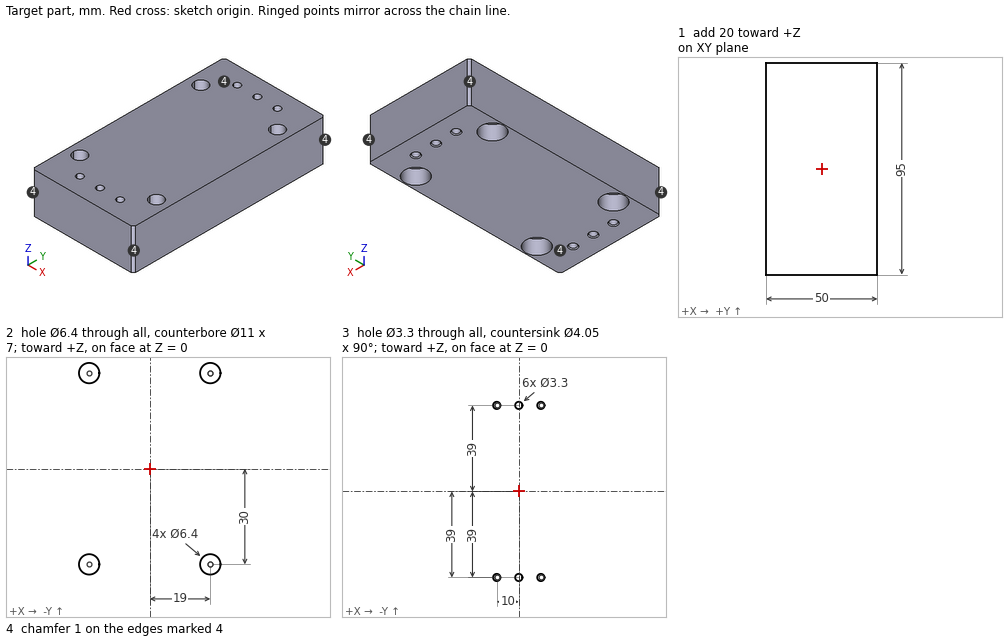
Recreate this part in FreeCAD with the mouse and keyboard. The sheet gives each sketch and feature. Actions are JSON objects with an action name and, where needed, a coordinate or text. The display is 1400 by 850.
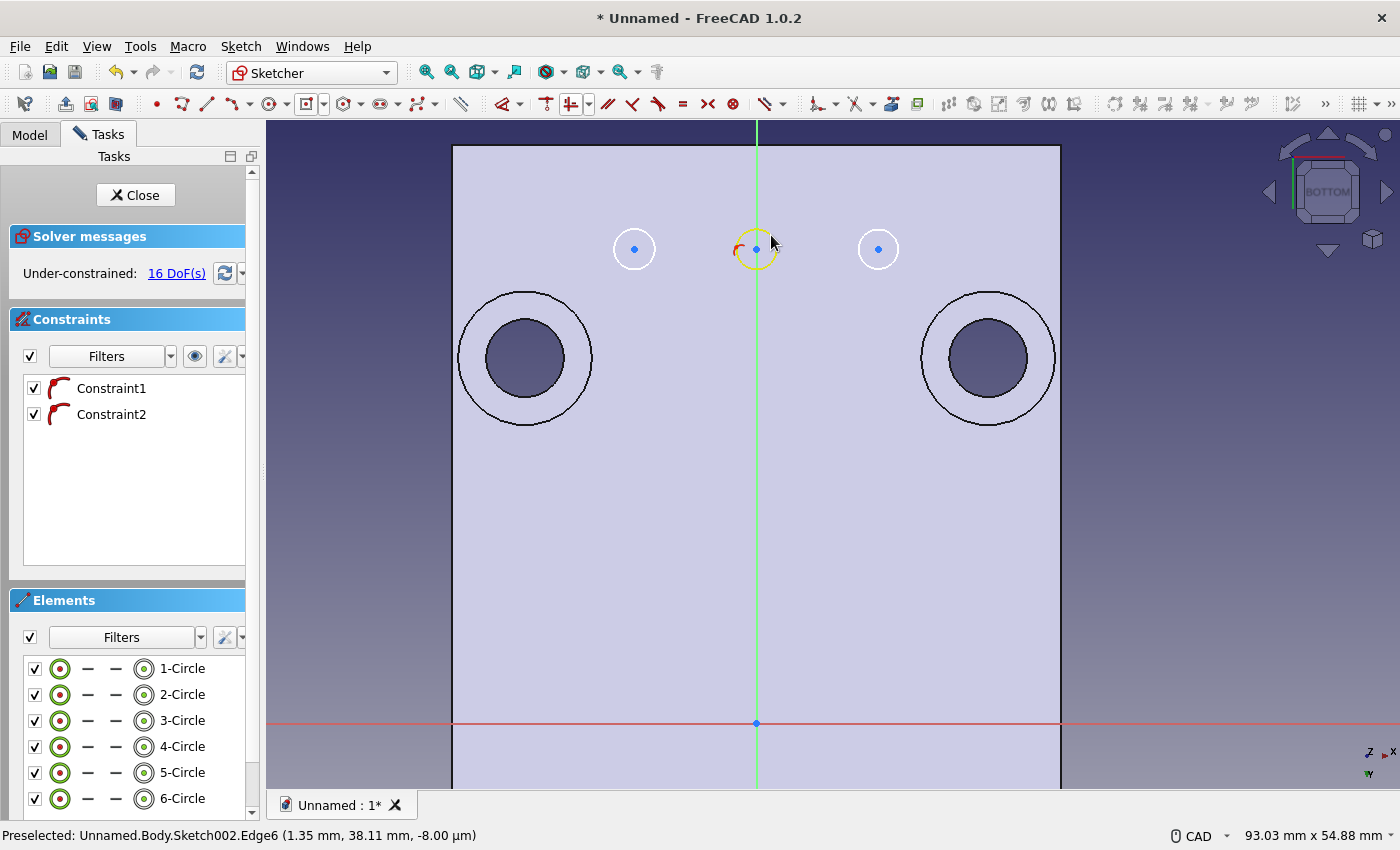
{"action": "left_click", "coordinate": [771, 235]}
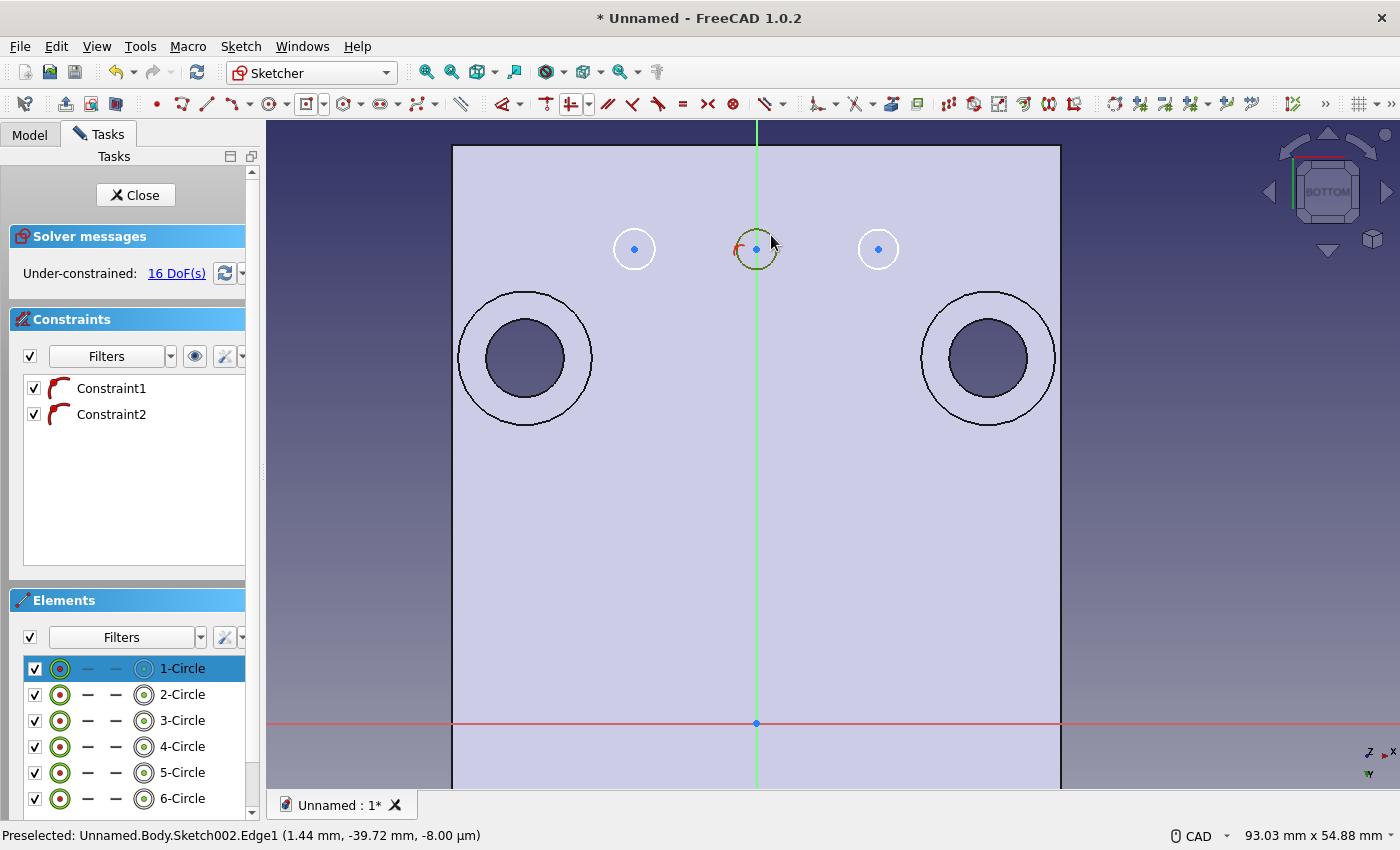
{"action": "scroll", "coordinate": [771, 235], "scroll_direction": "down", "scroll_amount": 4}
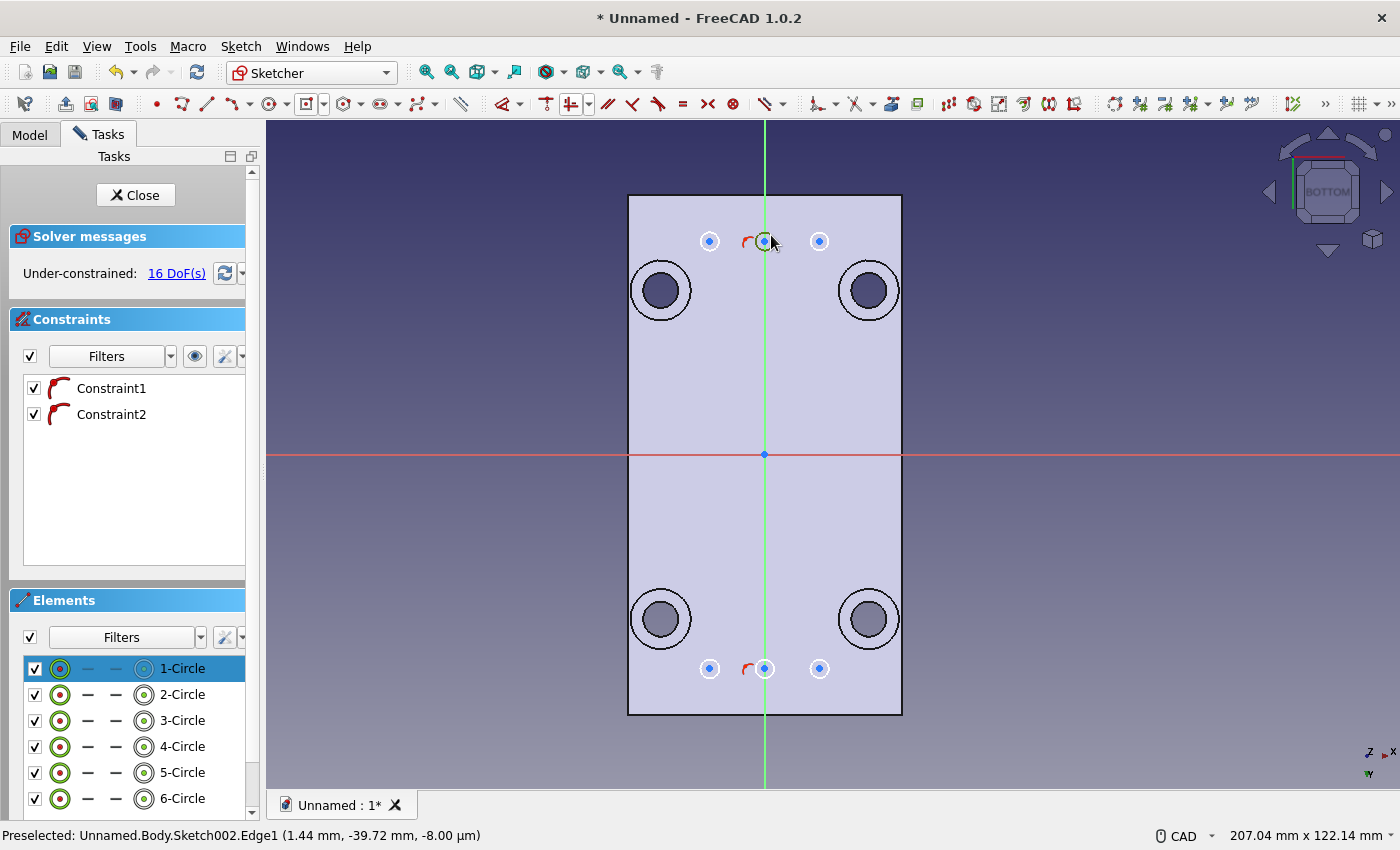
{"action": "scroll", "coordinate": [716, 662], "scroll_direction": "up", "scroll_amount": 2}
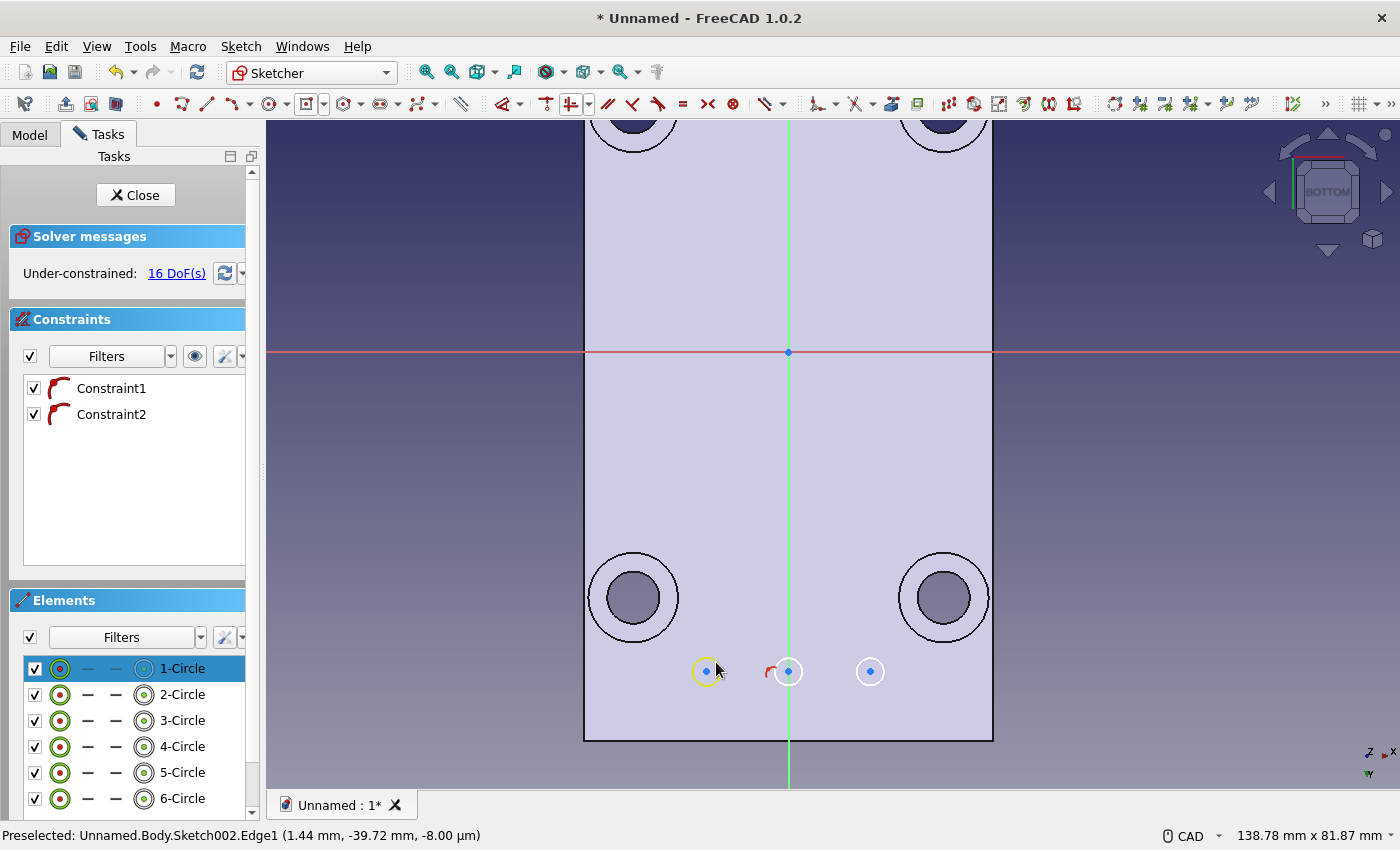
{"action": "left_click", "coordinate": [717, 662]}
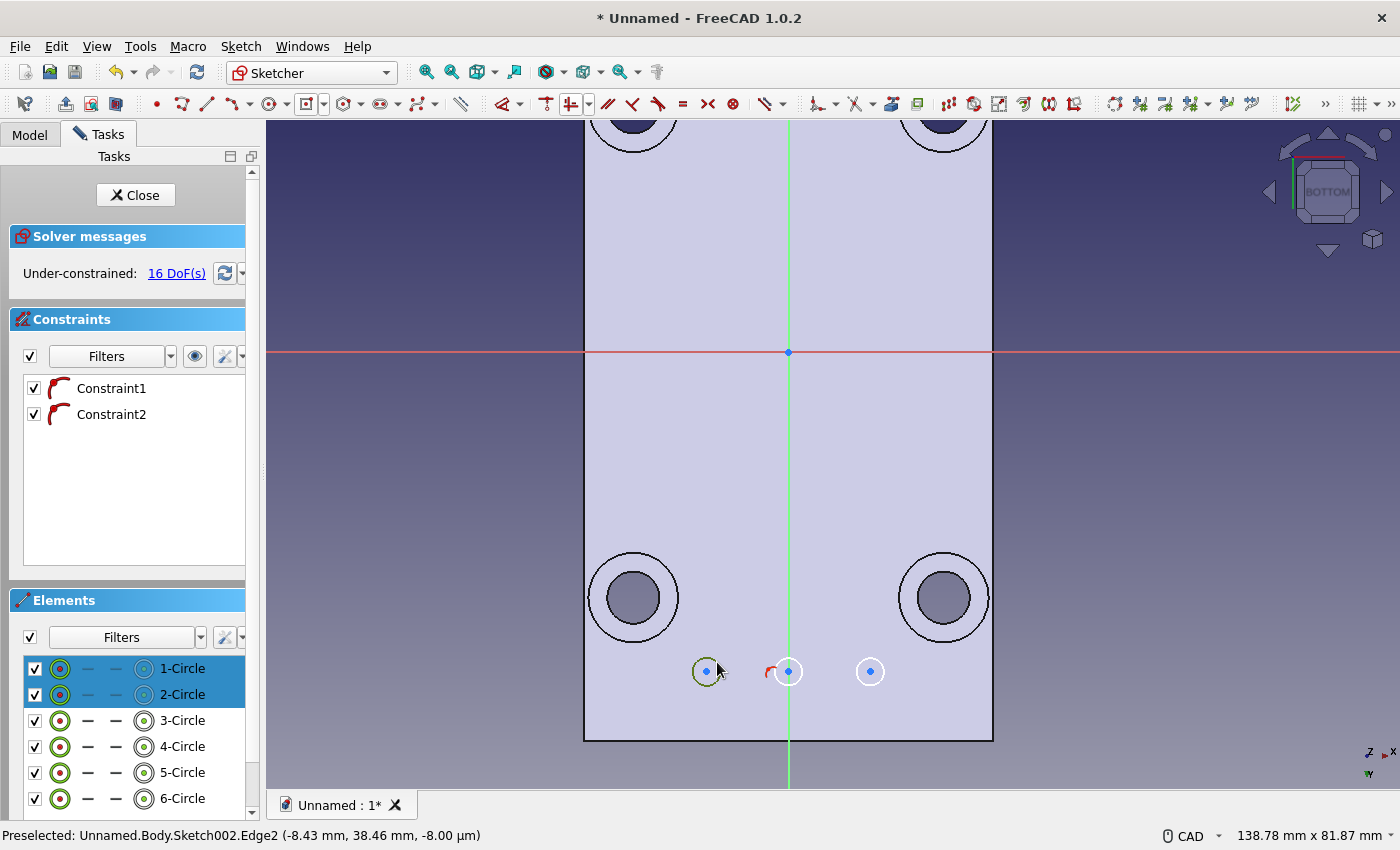
{"action": "scroll", "coordinate": [716, 662], "scroll_direction": "down", "scroll_amount": 2}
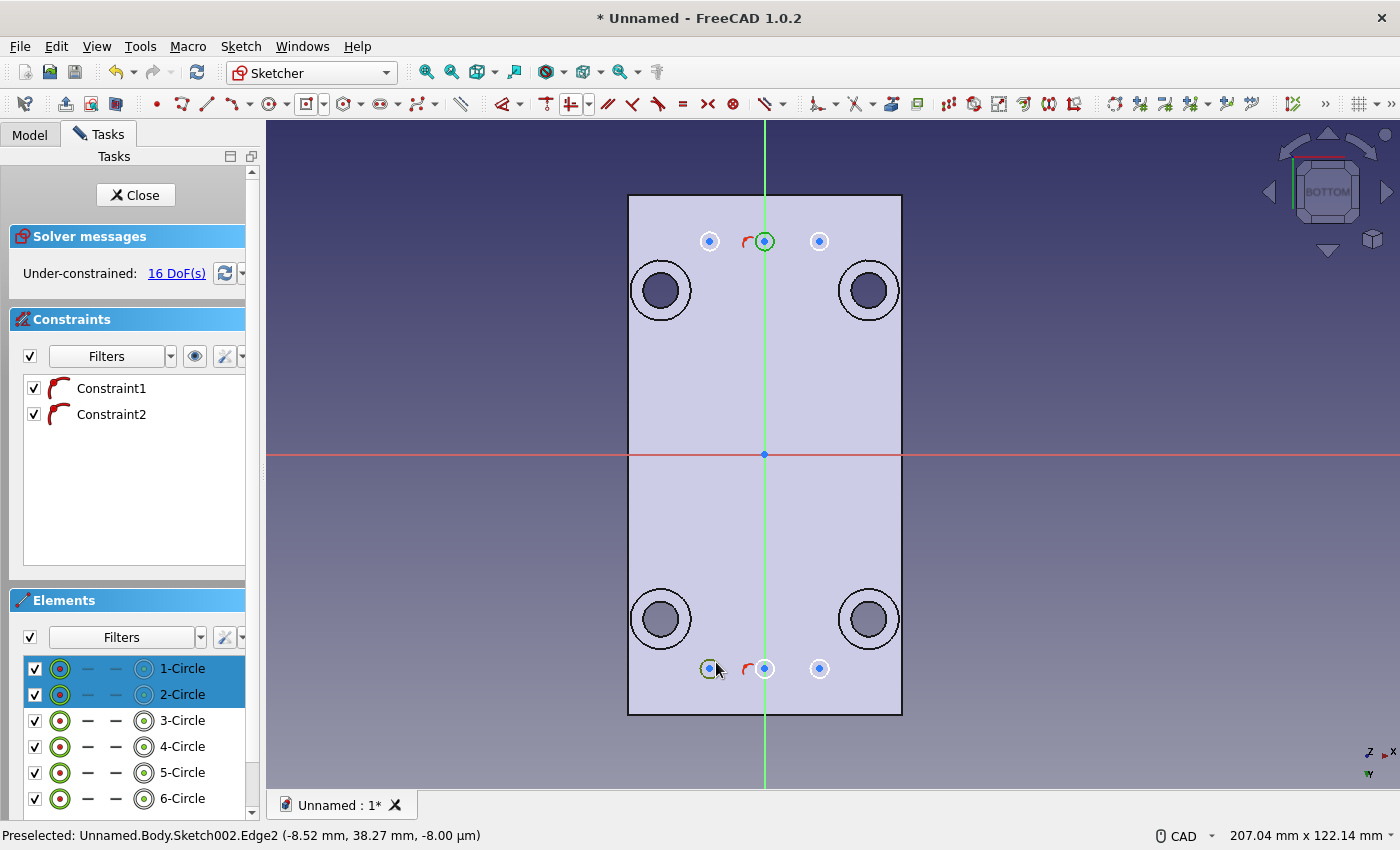
{"action": "scroll", "coordinate": [716, 235], "scroll_direction": "up", "scroll_amount": 3}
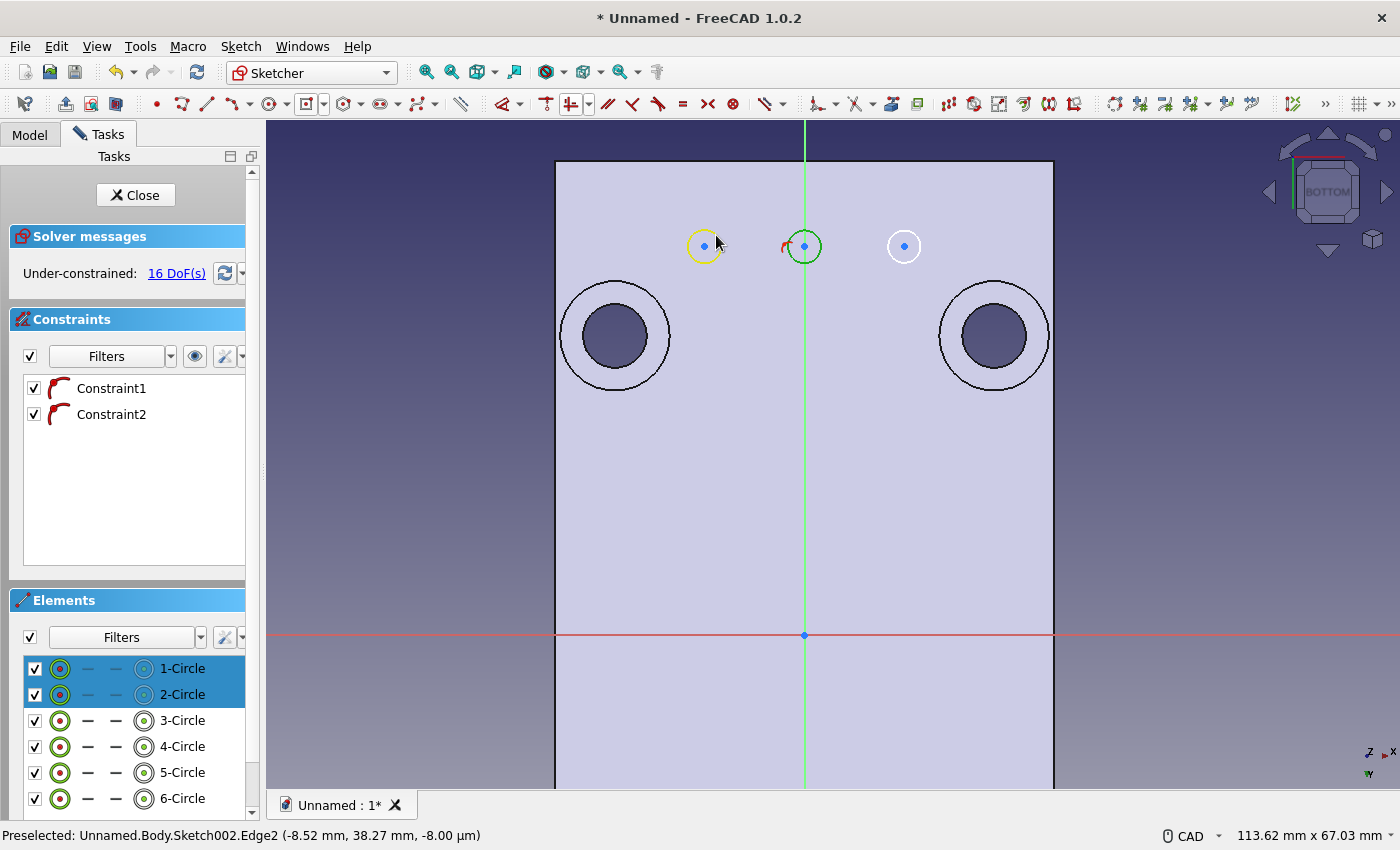
{"action": "left_click", "coordinate": [716, 235]}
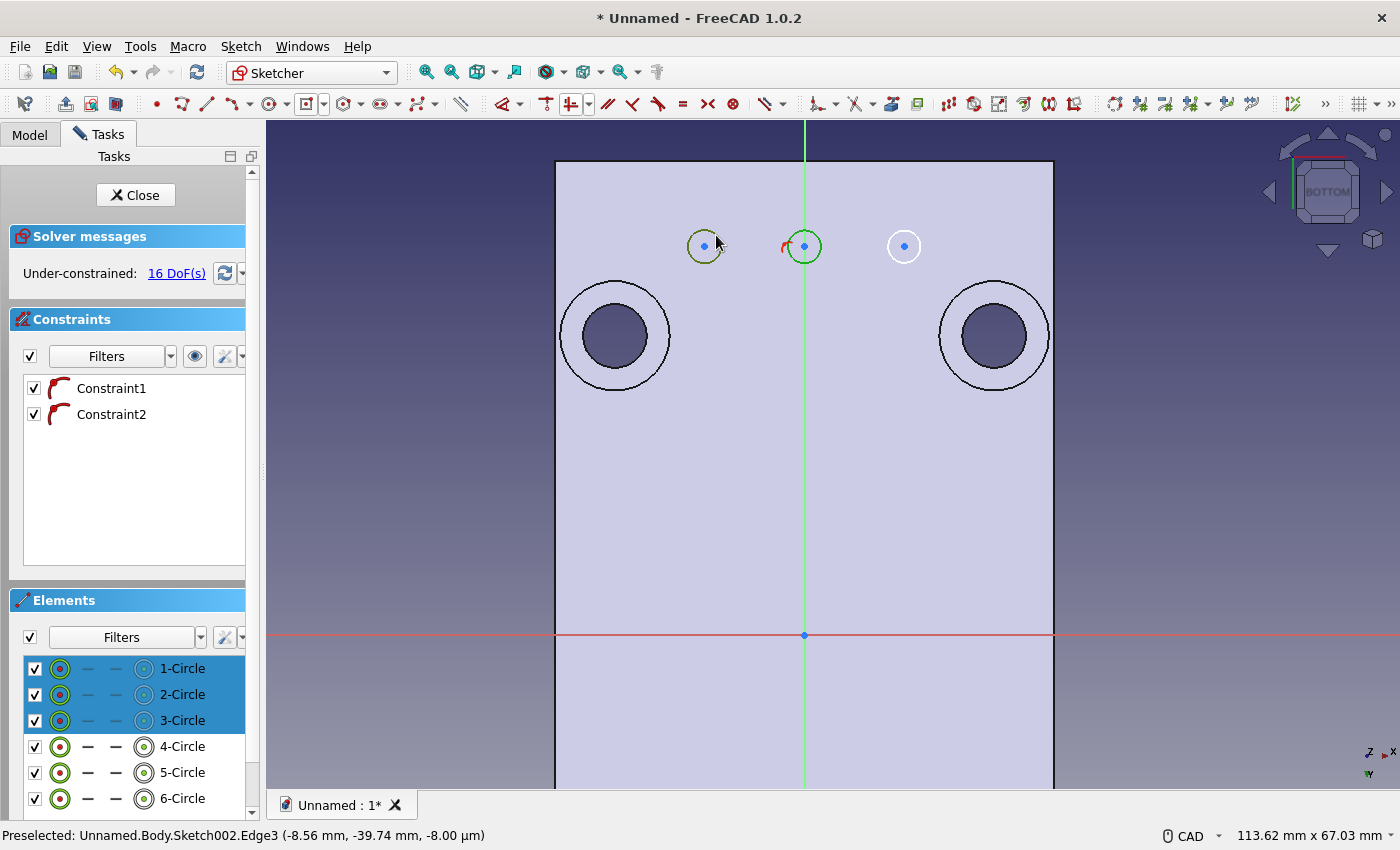
{"action": "left_click", "coordinate": [916, 235]}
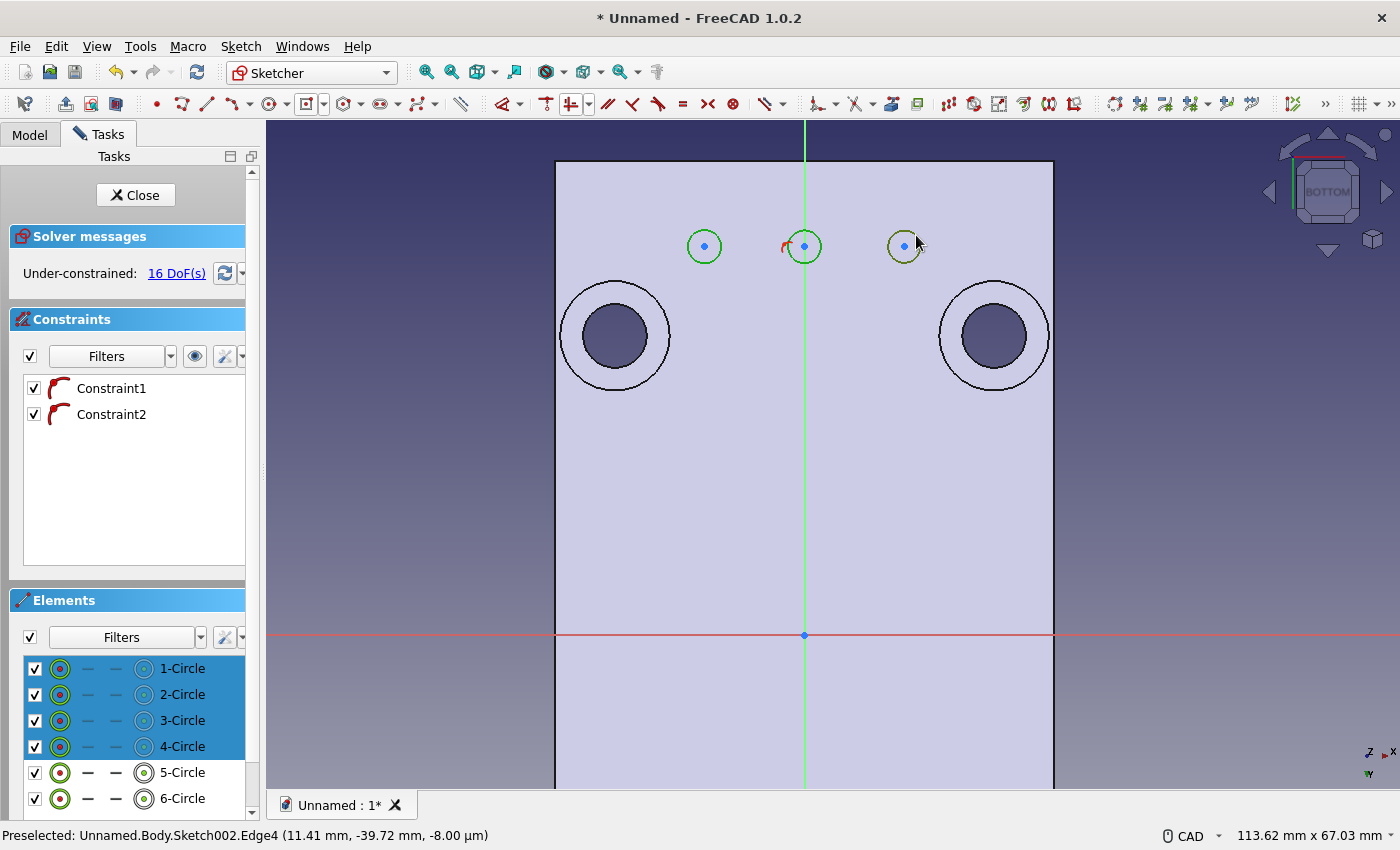
{"action": "scroll", "coordinate": [716, 235], "scroll_direction": "down", "scroll_amount": 3}